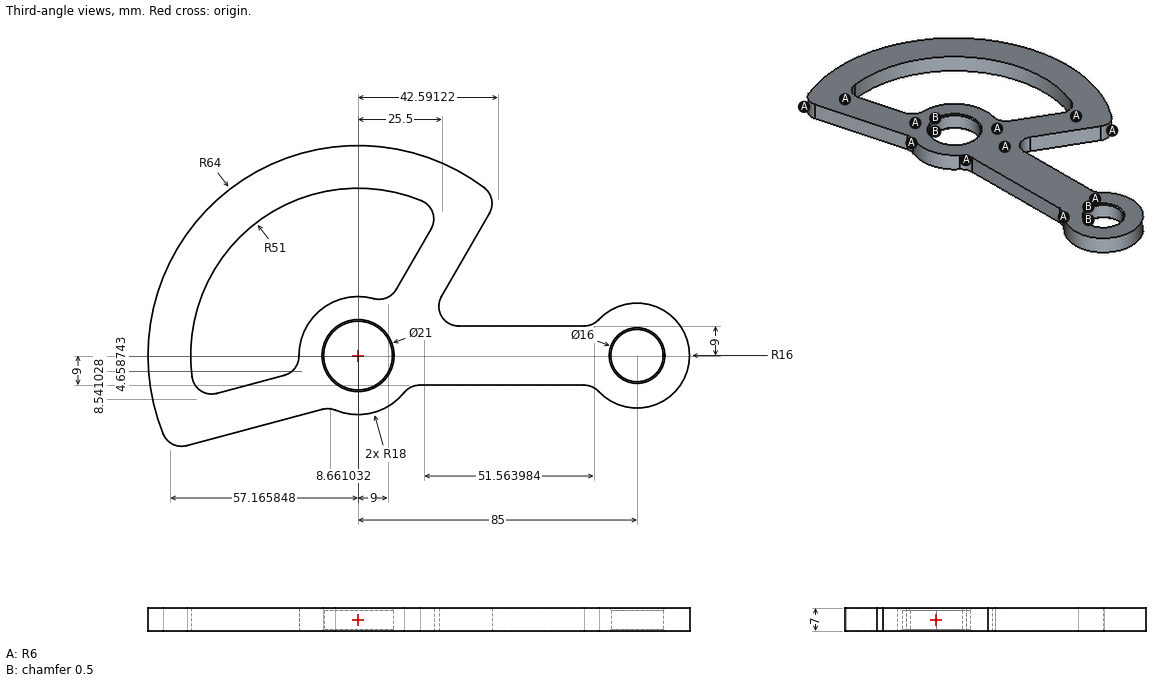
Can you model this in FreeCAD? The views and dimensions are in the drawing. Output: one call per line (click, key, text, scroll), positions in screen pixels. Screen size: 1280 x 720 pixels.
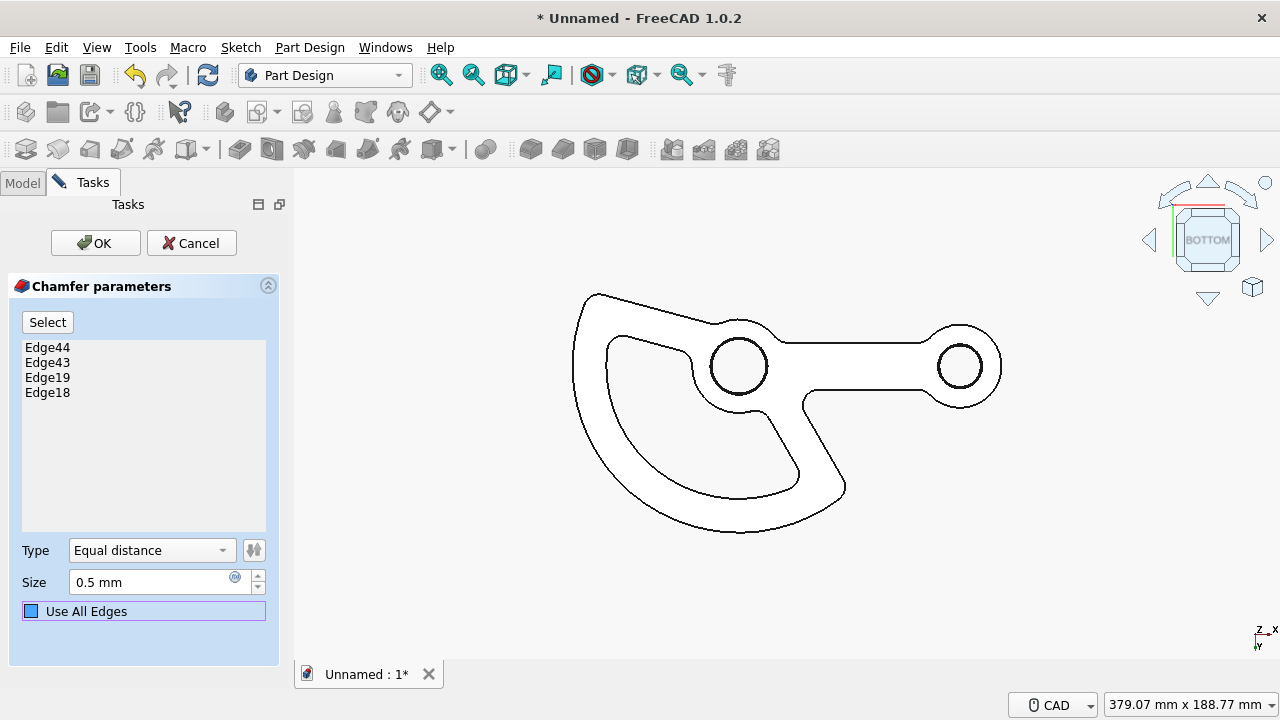
click(96, 243)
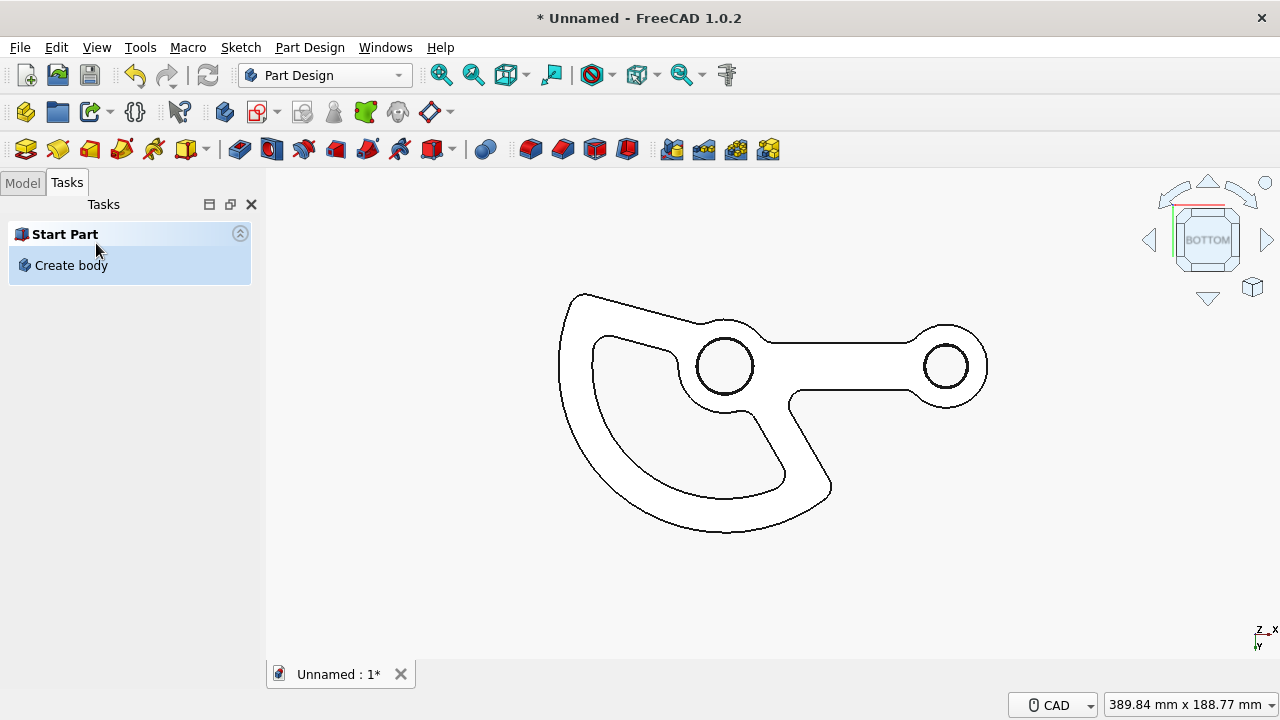
key(0)